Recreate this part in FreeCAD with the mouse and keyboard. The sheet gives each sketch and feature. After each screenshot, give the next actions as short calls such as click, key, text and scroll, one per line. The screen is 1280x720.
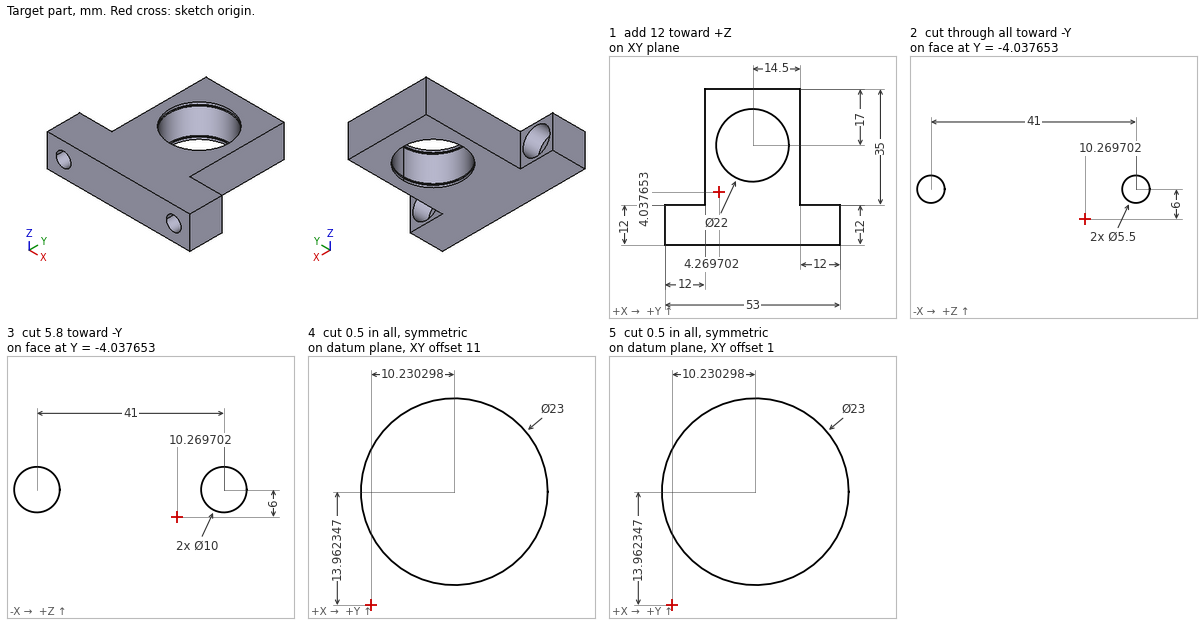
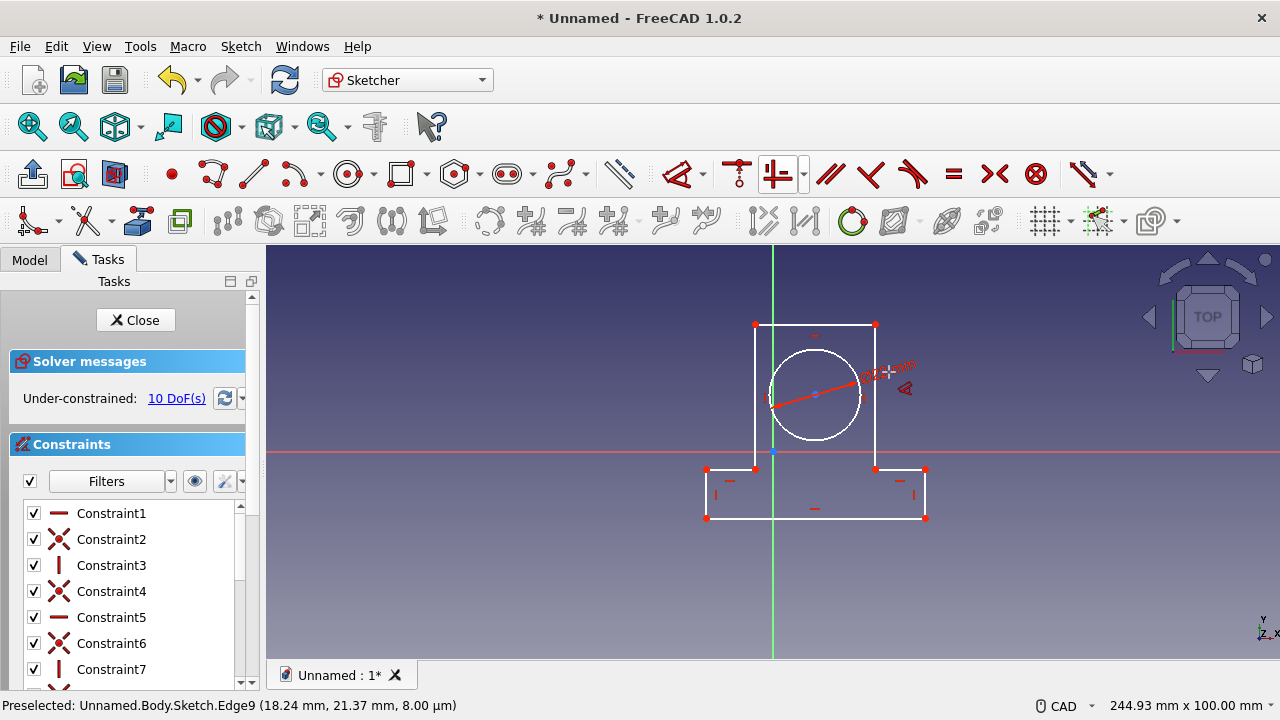
click(740, 470)
click(730, 504)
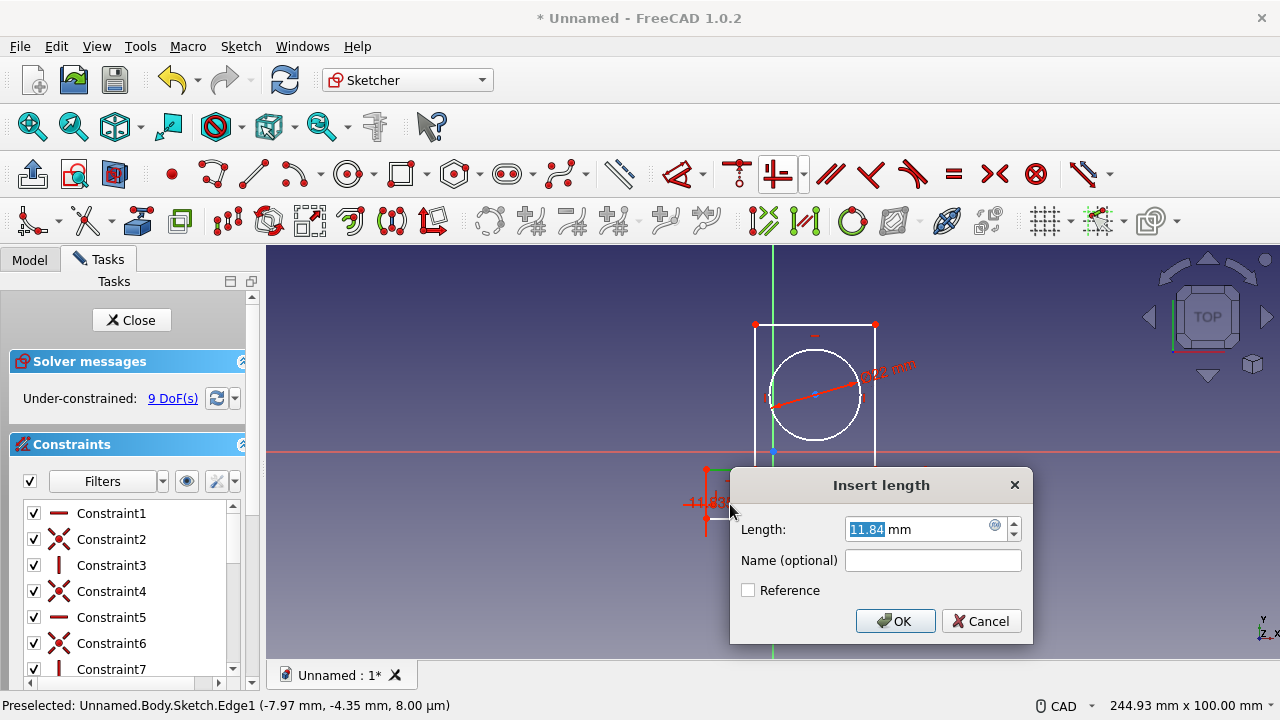
text(12)
key(Return)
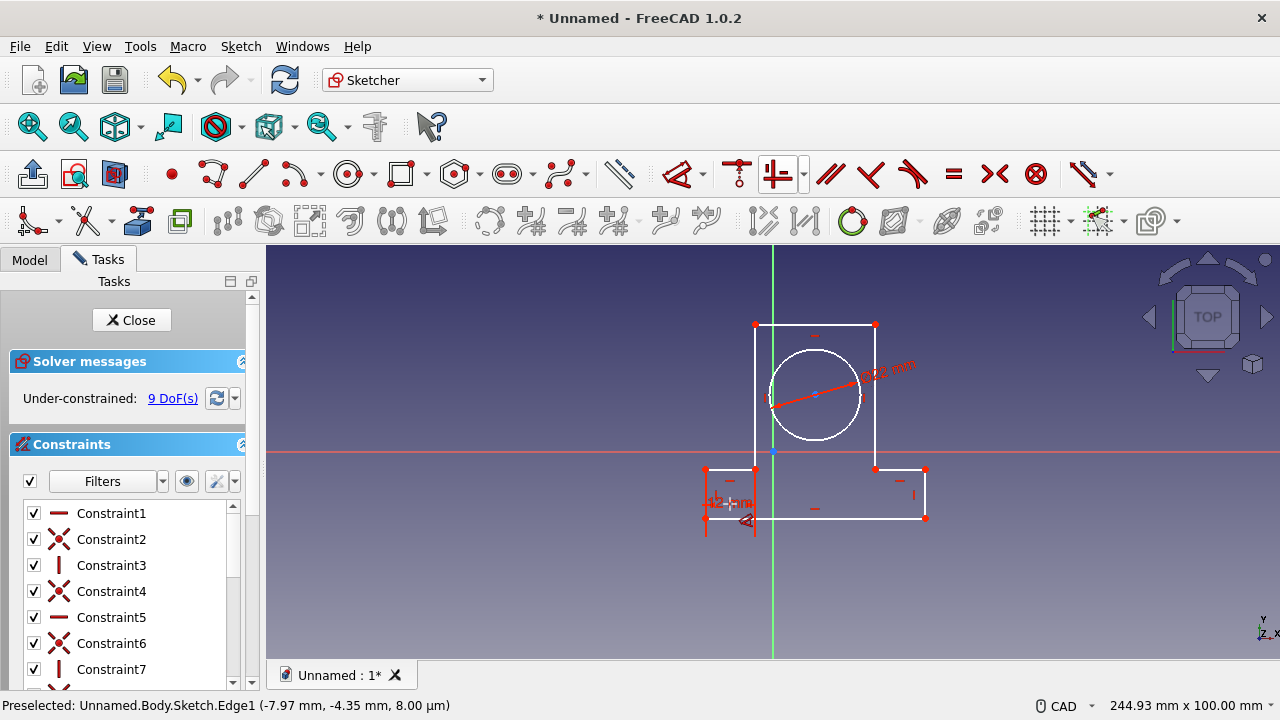
click(706, 485)
click(672, 483)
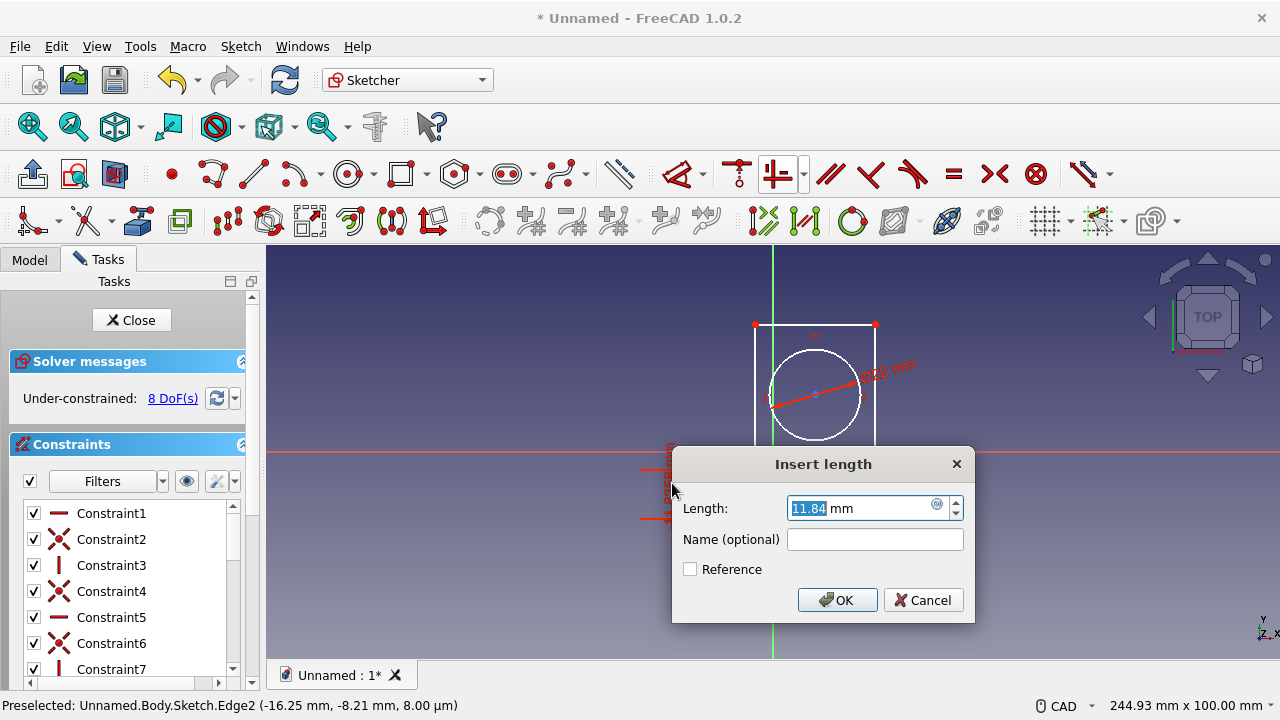
text(12)
key(Return)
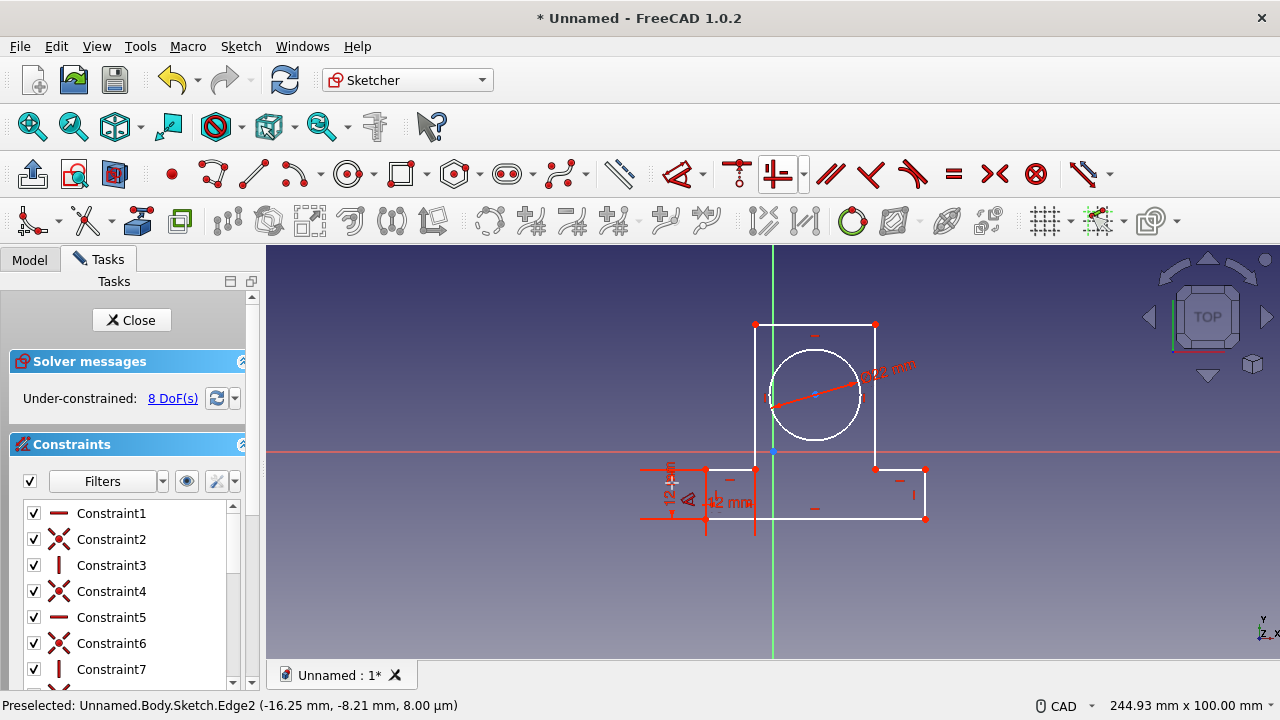
click(771, 519)
click(815, 553)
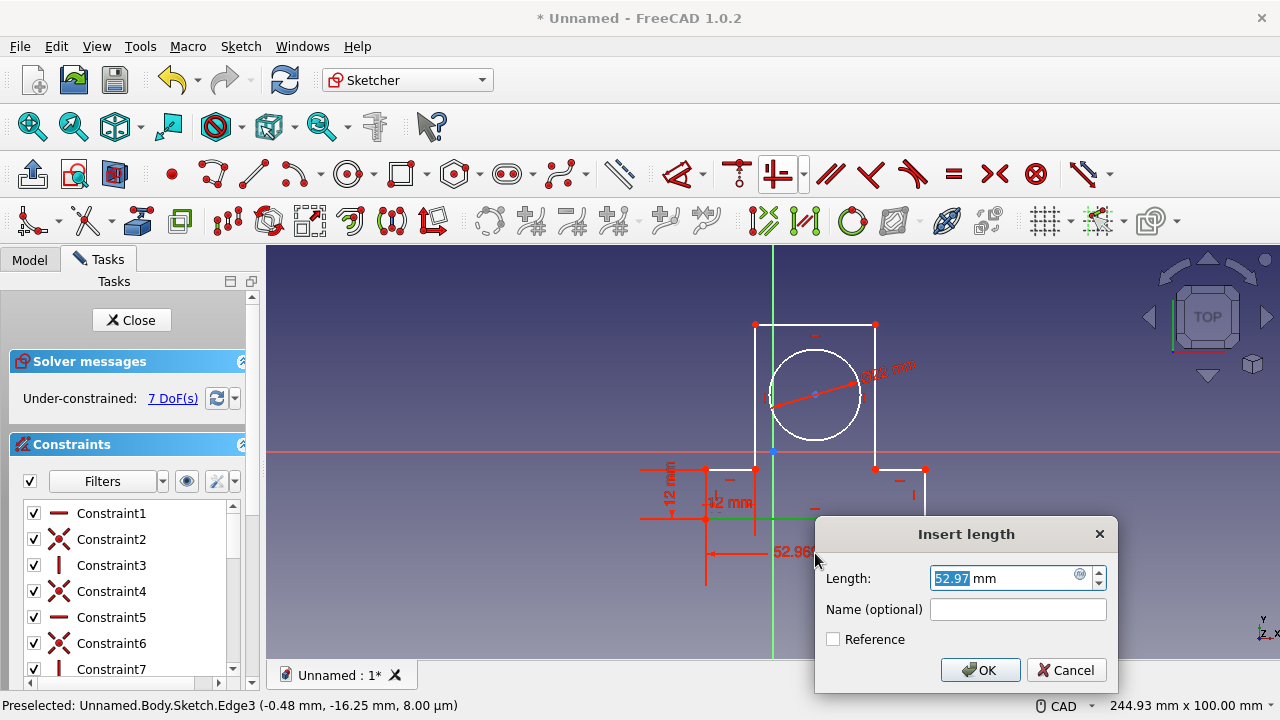
text(53)
key(Return)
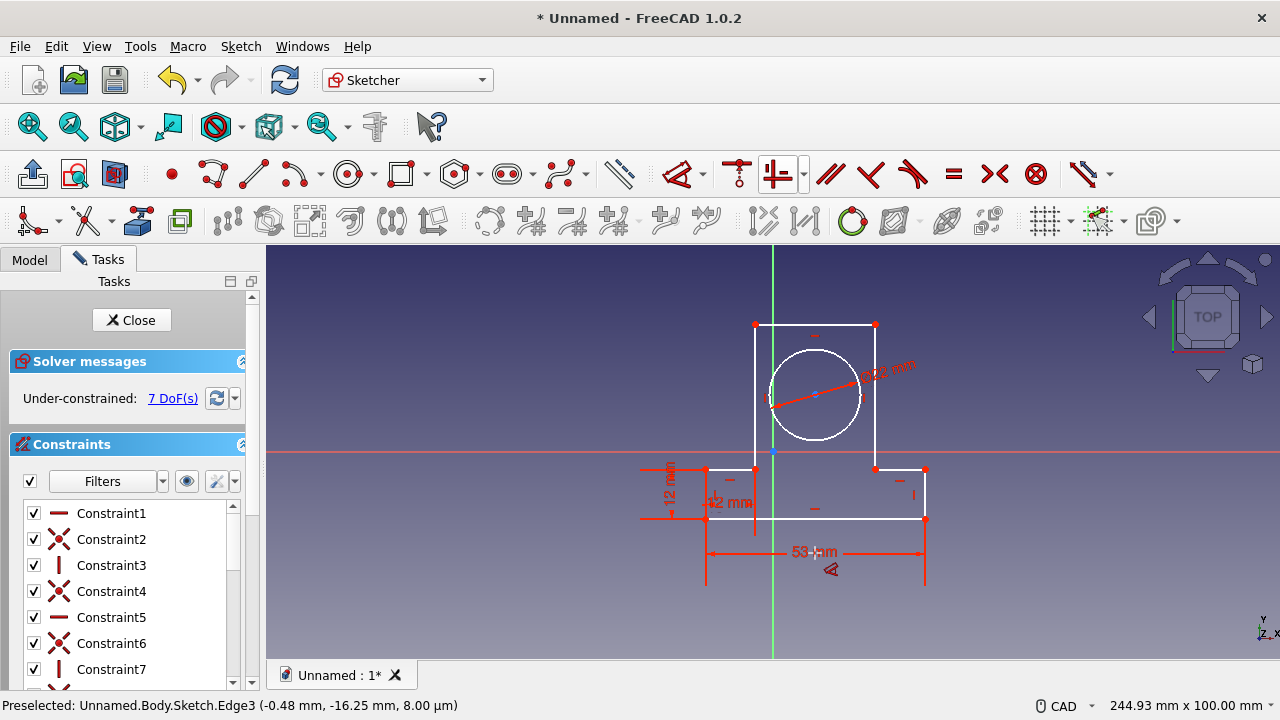
click(925, 505)
click(959, 495)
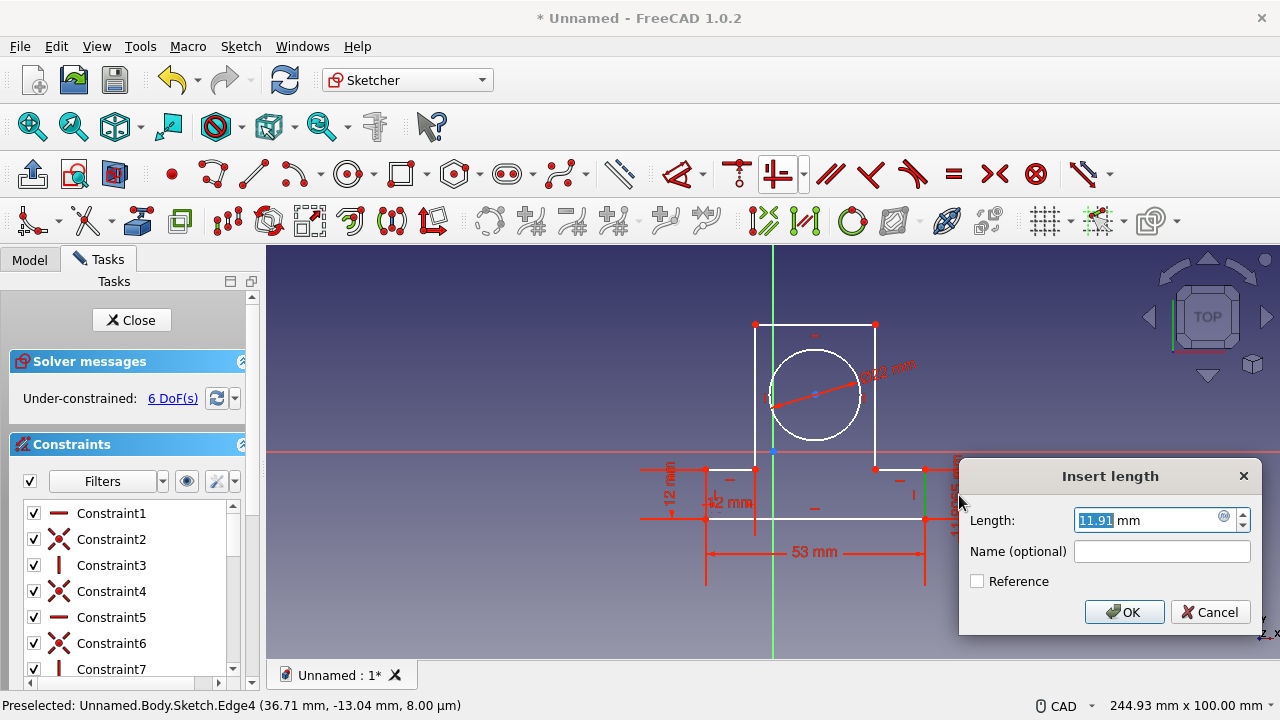
text(12)
key(Return)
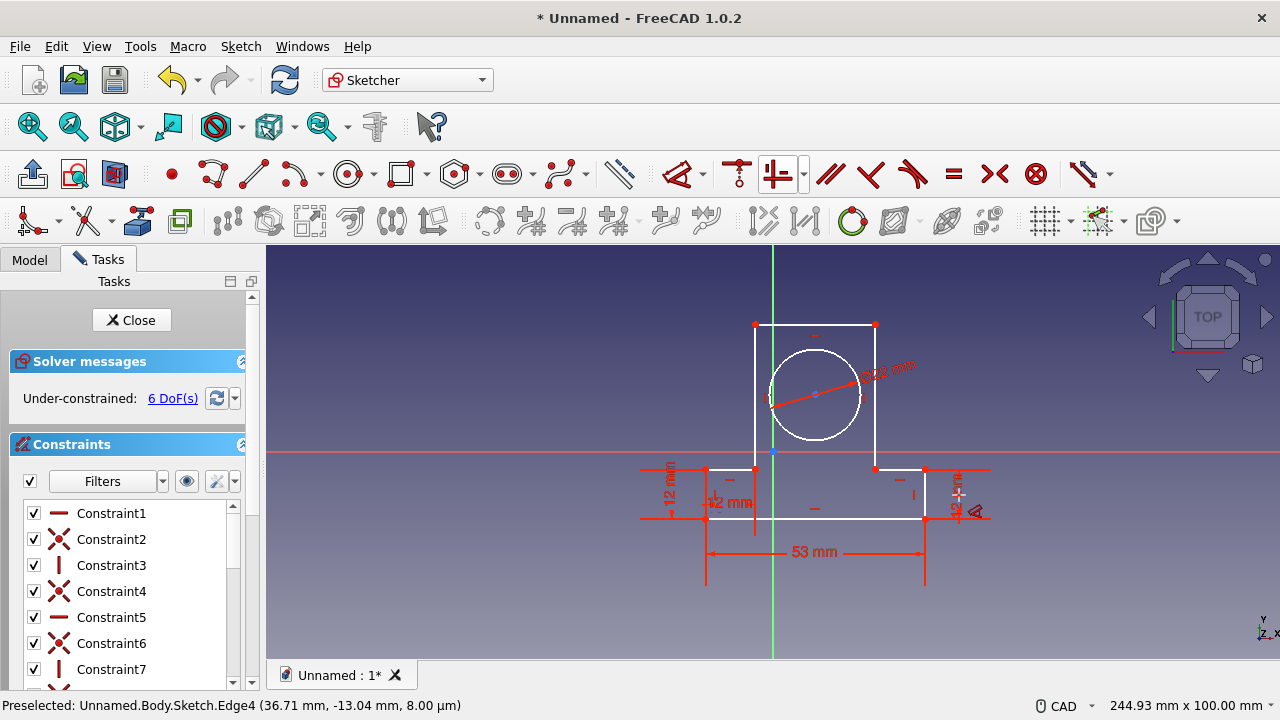
click(910, 470)
click(889, 504)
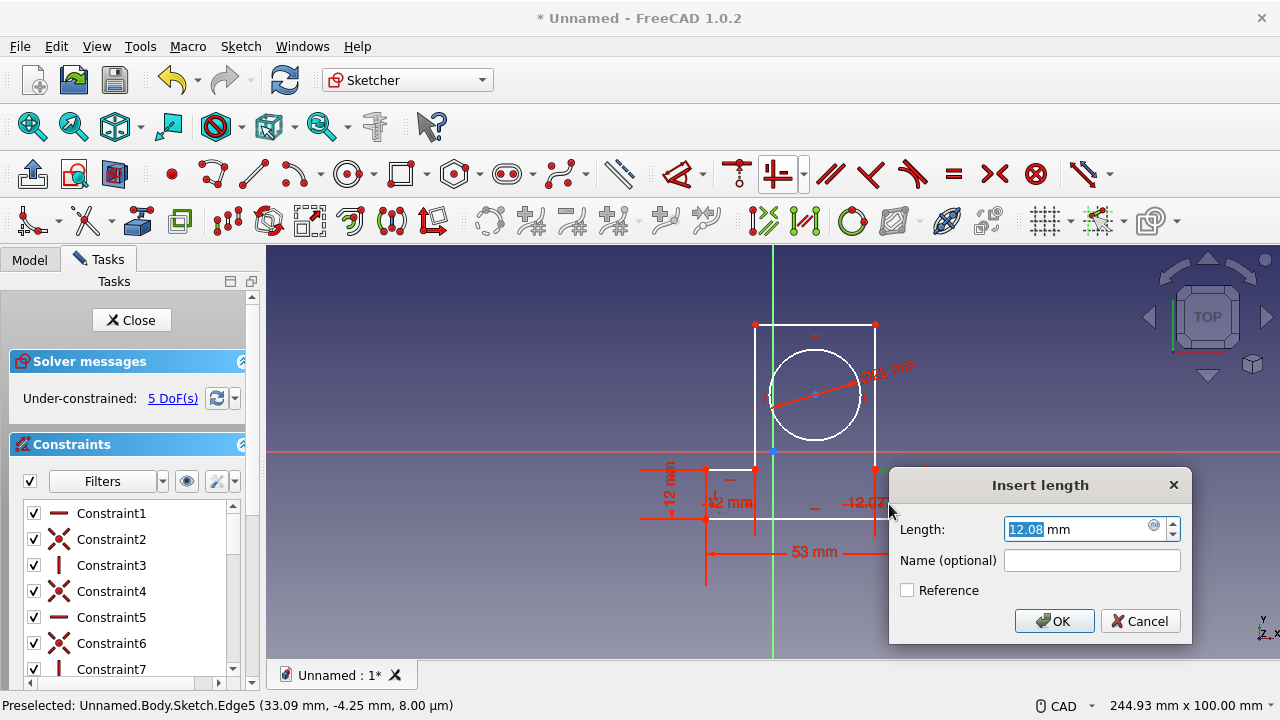
text(12)
key(Return)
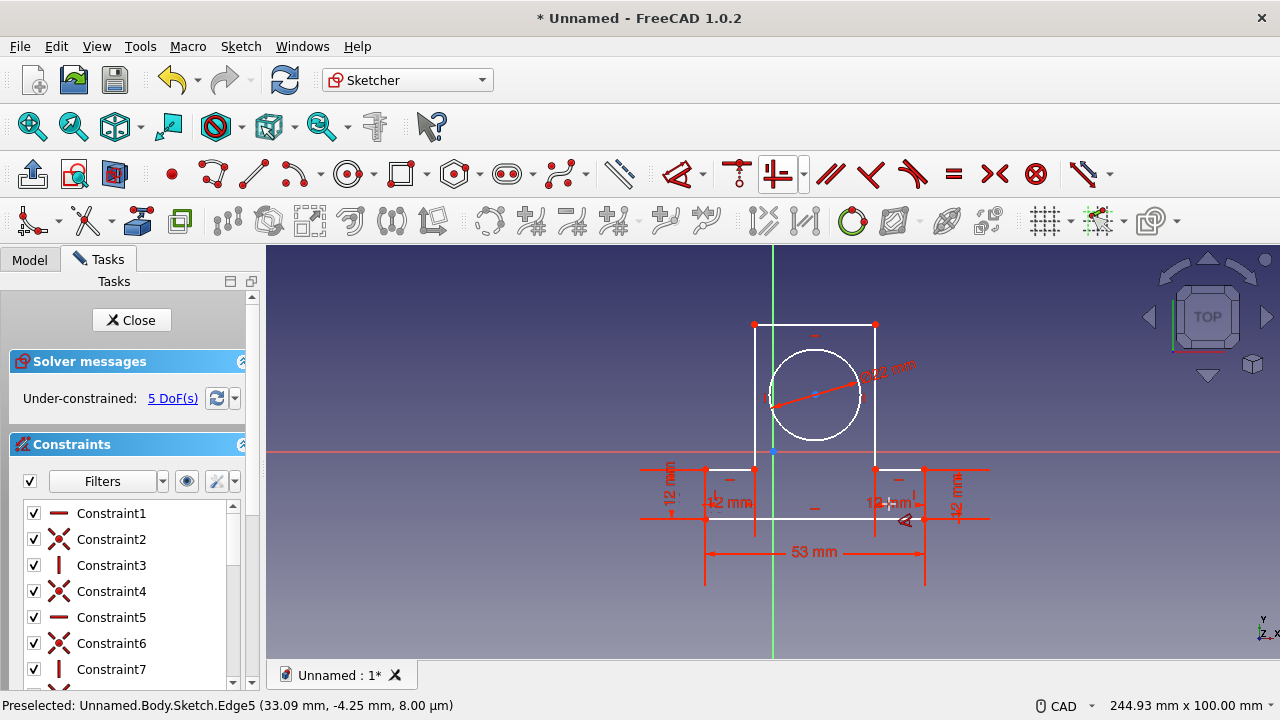
click(875, 426)
click(909, 397)